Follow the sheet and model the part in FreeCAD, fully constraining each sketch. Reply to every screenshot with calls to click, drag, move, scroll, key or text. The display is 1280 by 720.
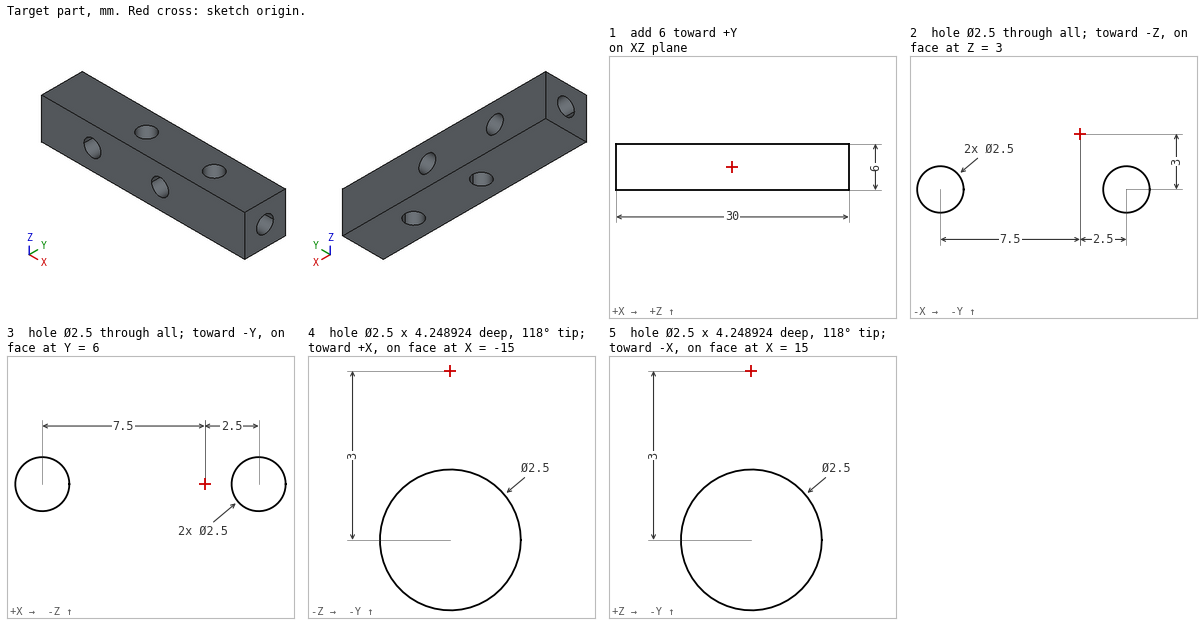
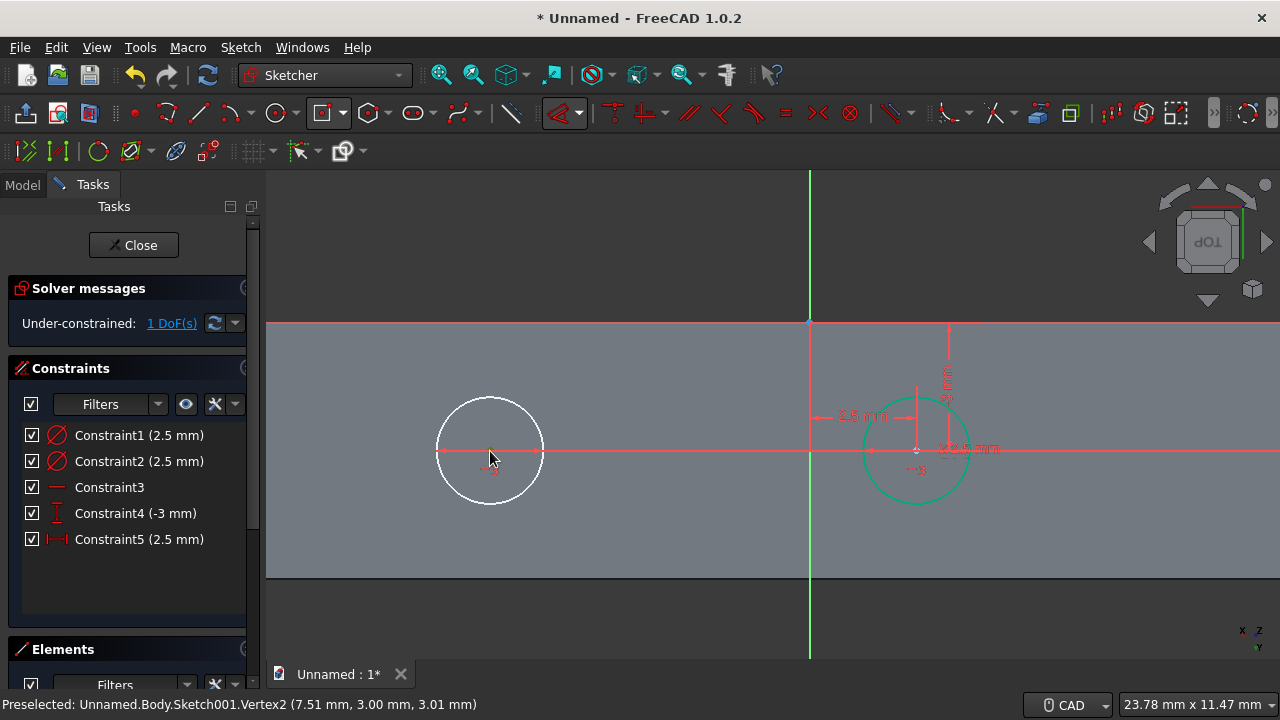
key(l)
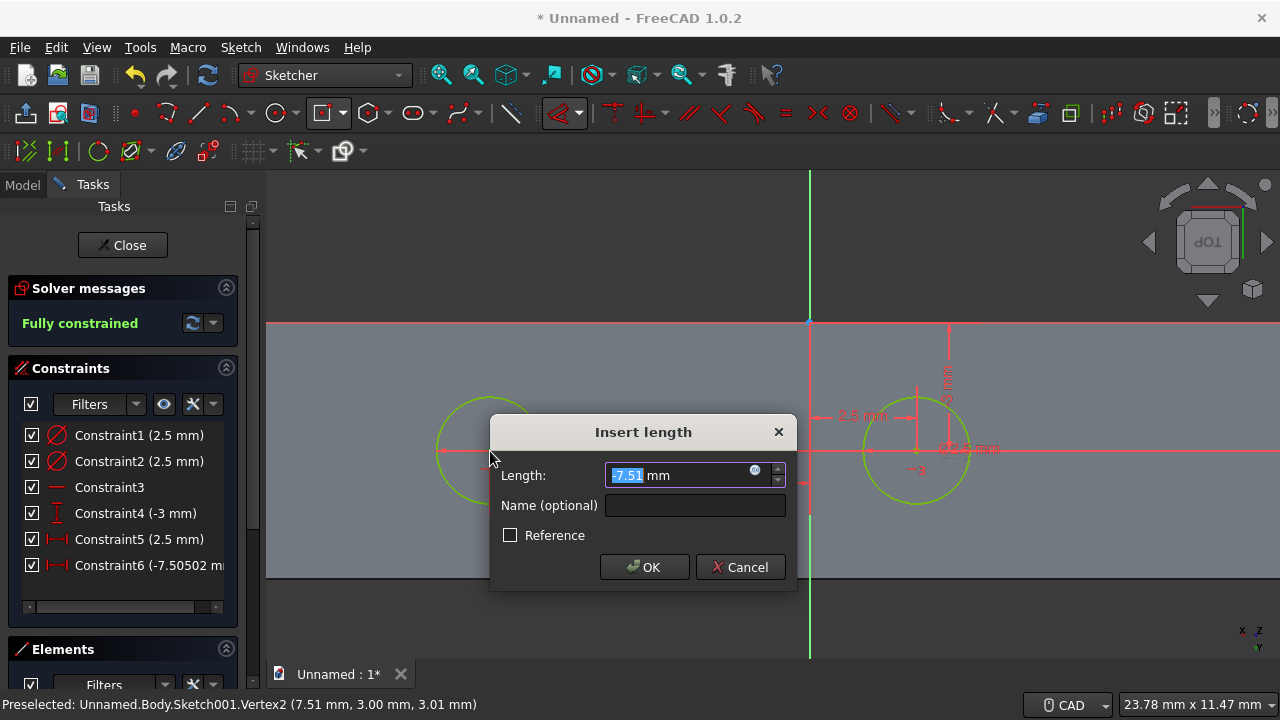
text(-7.5)
key(Return)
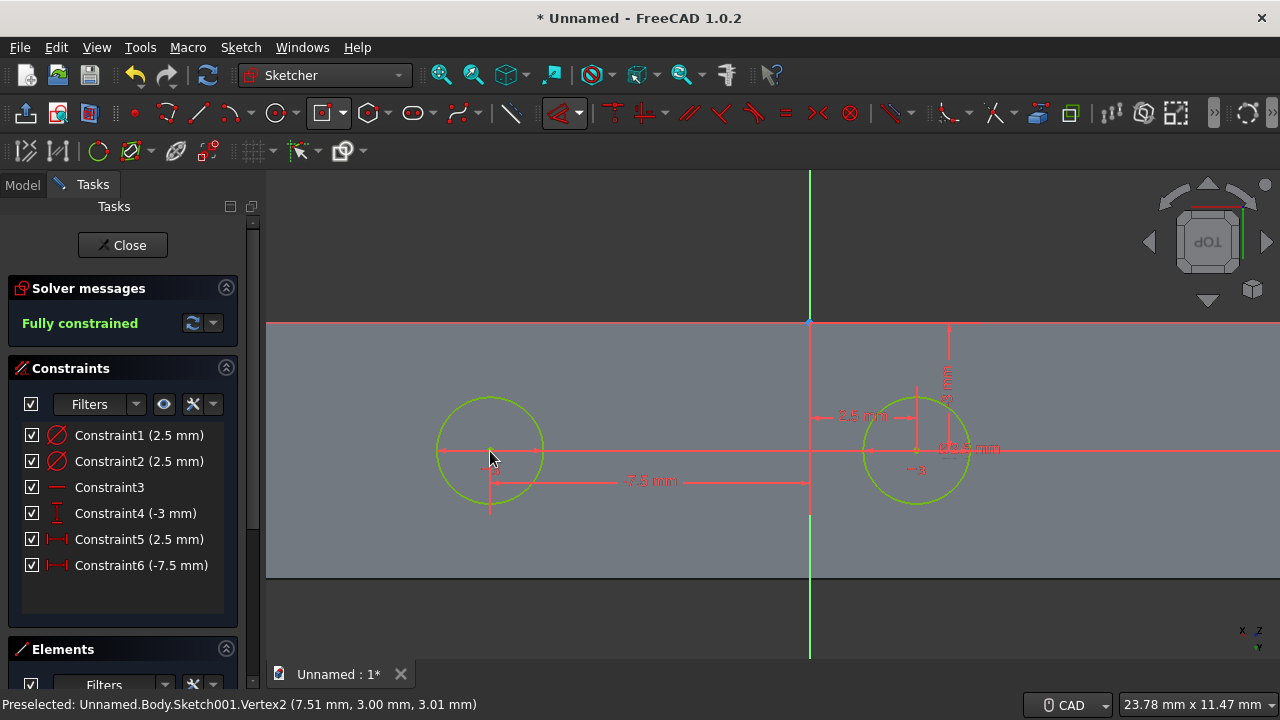
click(123, 245)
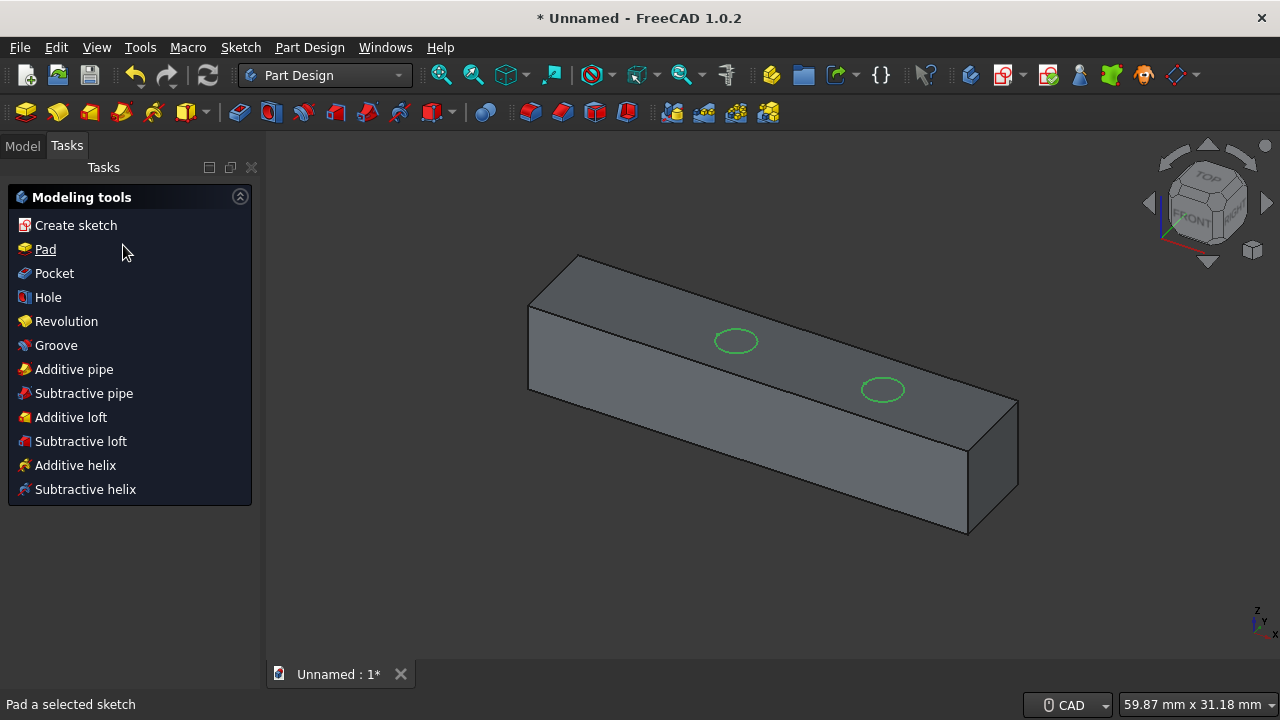
click(272, 112)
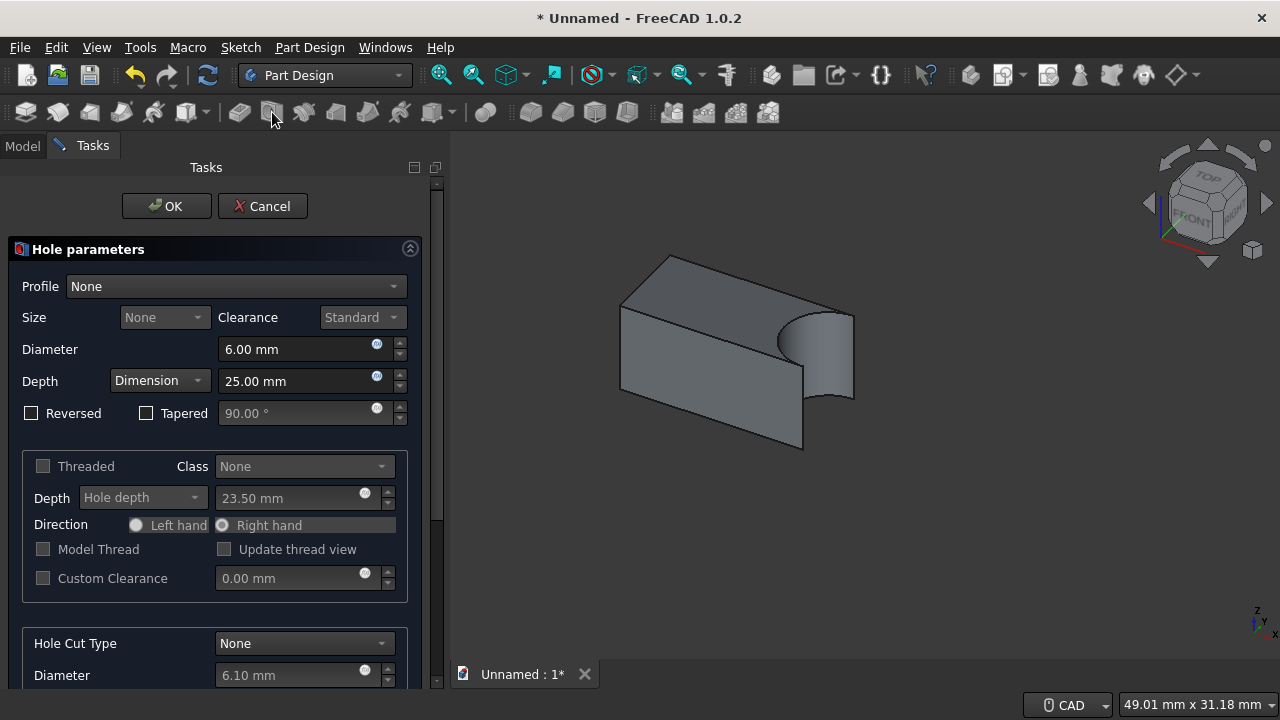
triple_click(305, 349)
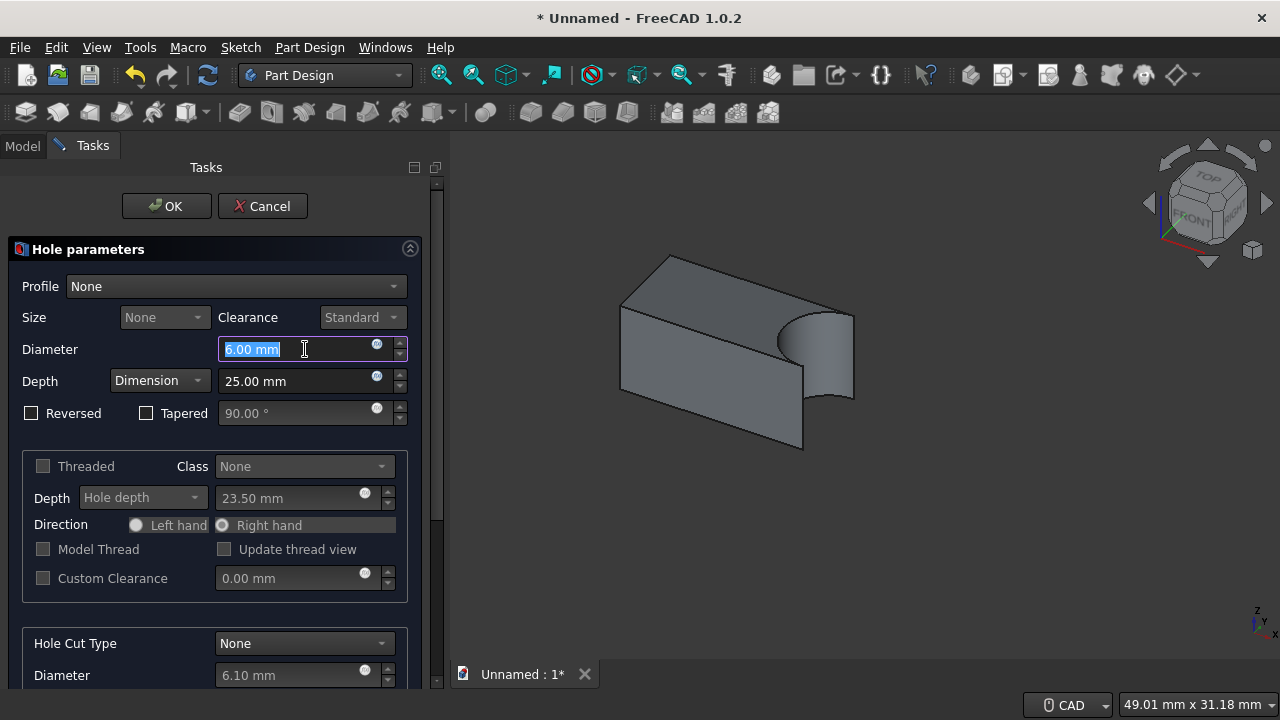
text(2.5)
key(Tab)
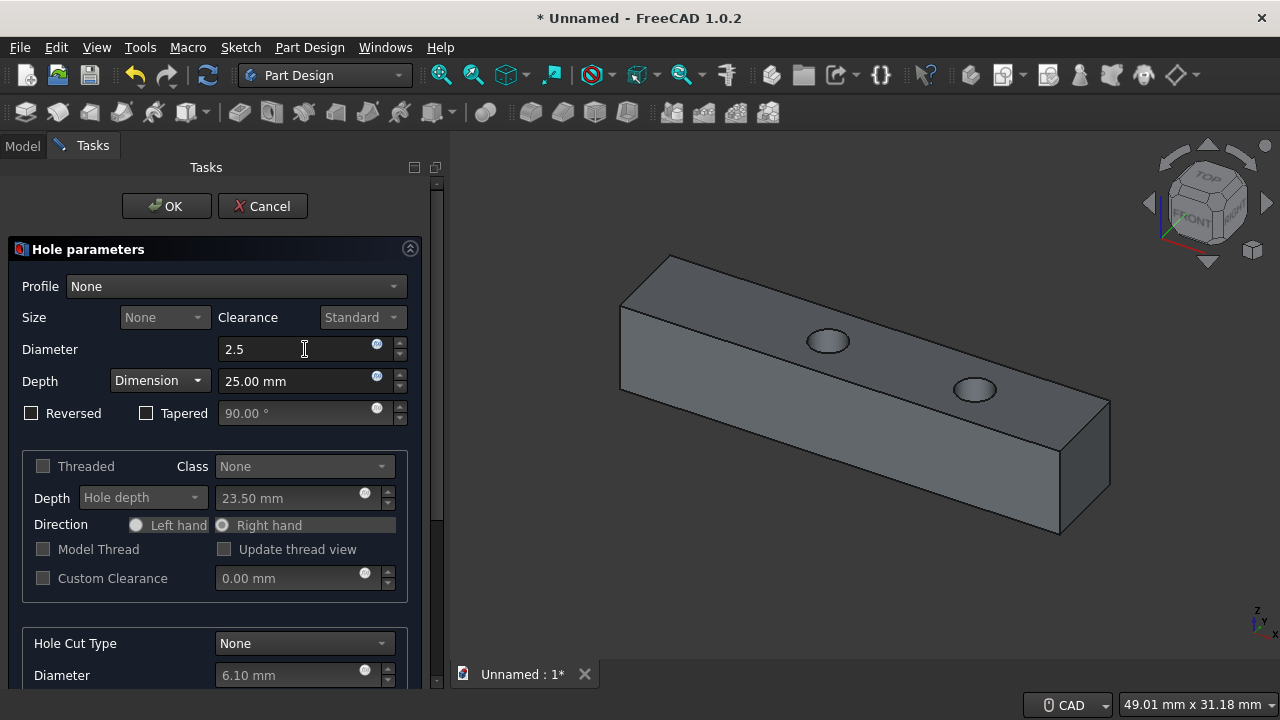
click(161, 380)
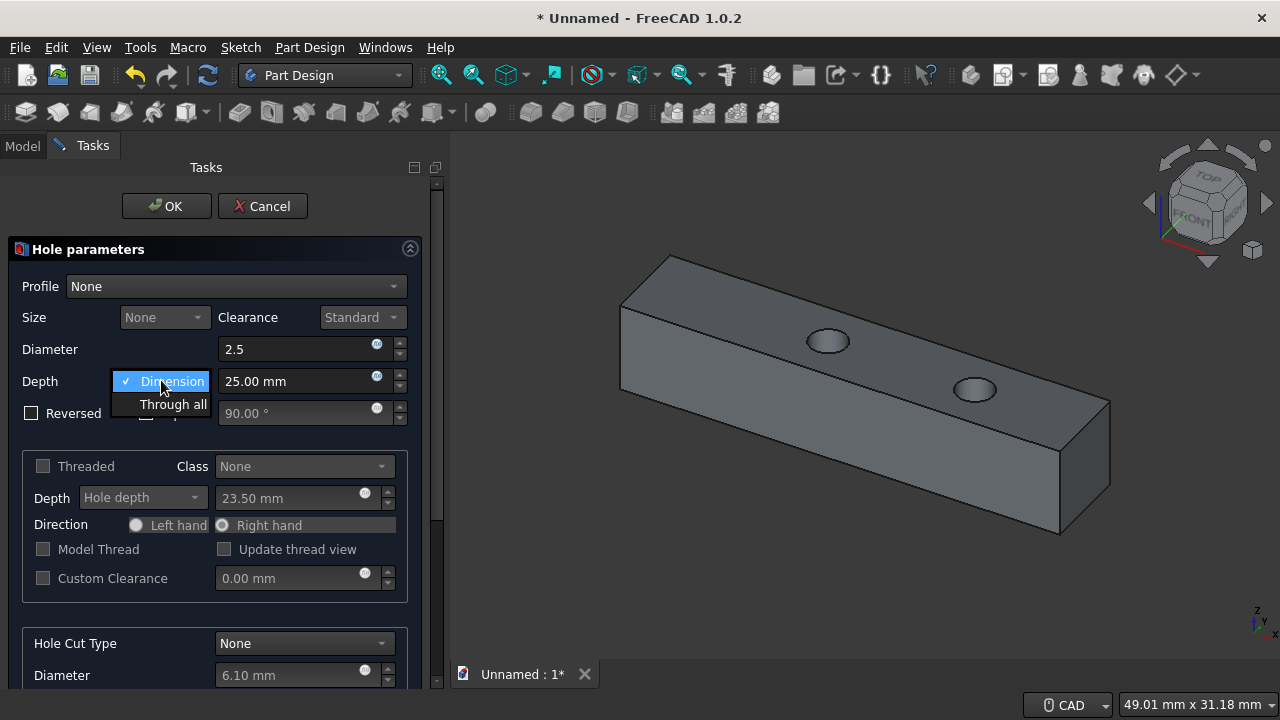
click(160, 404)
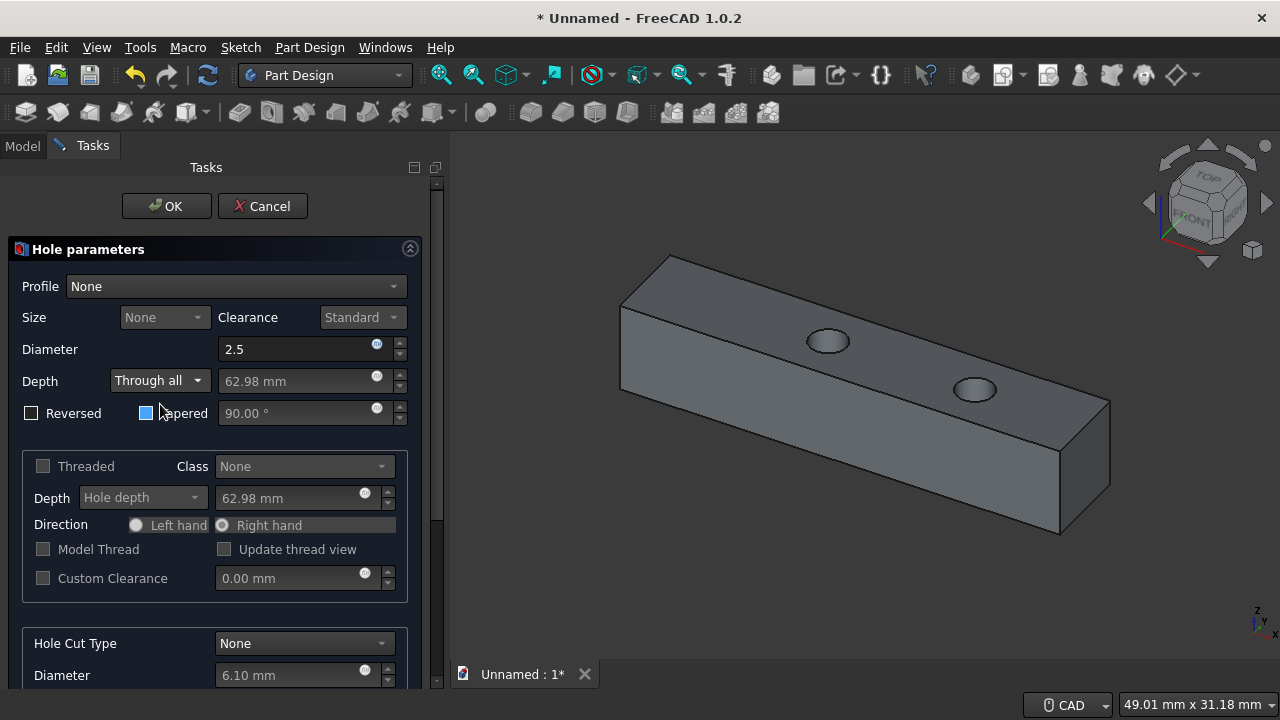
click(167, 206)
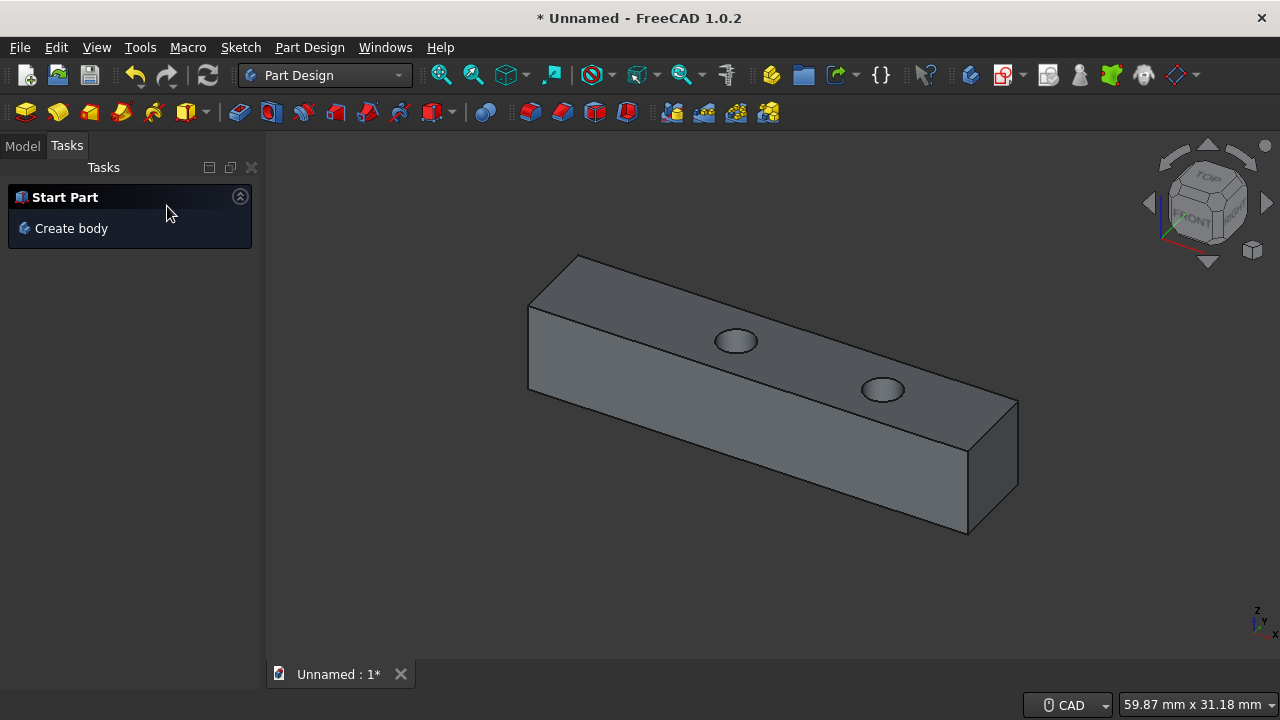
key(4)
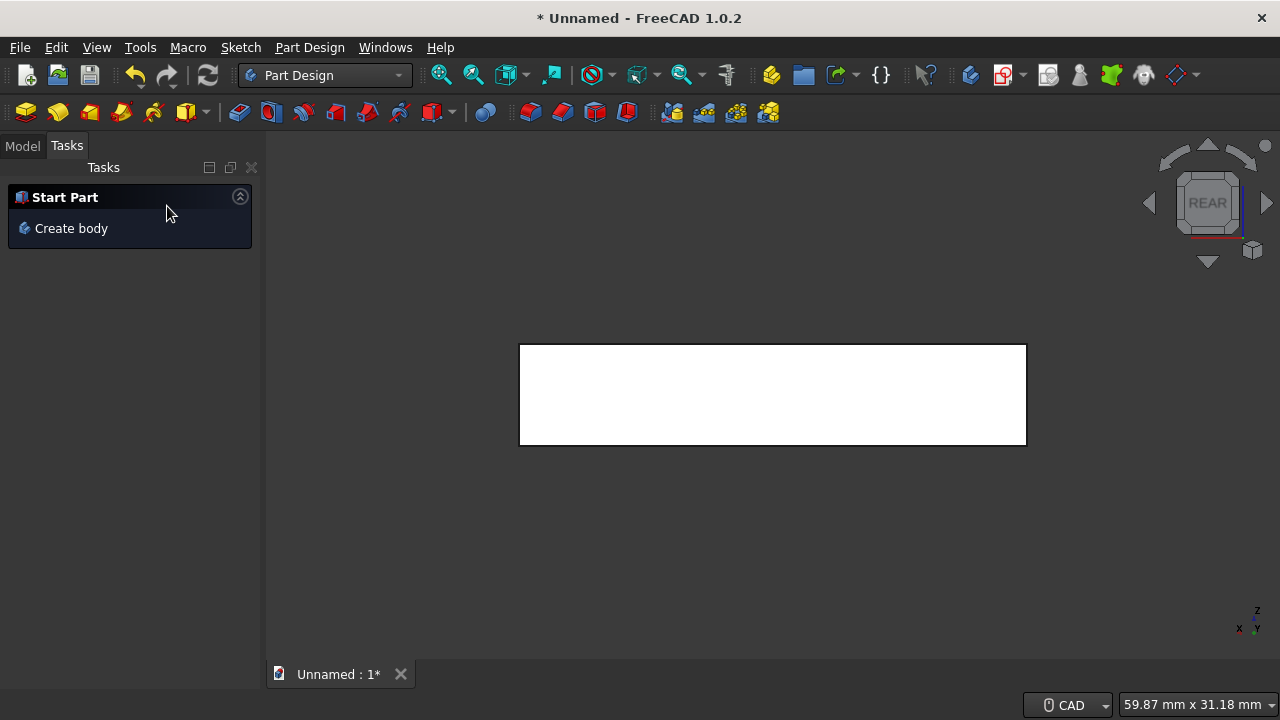
click(628, 394)